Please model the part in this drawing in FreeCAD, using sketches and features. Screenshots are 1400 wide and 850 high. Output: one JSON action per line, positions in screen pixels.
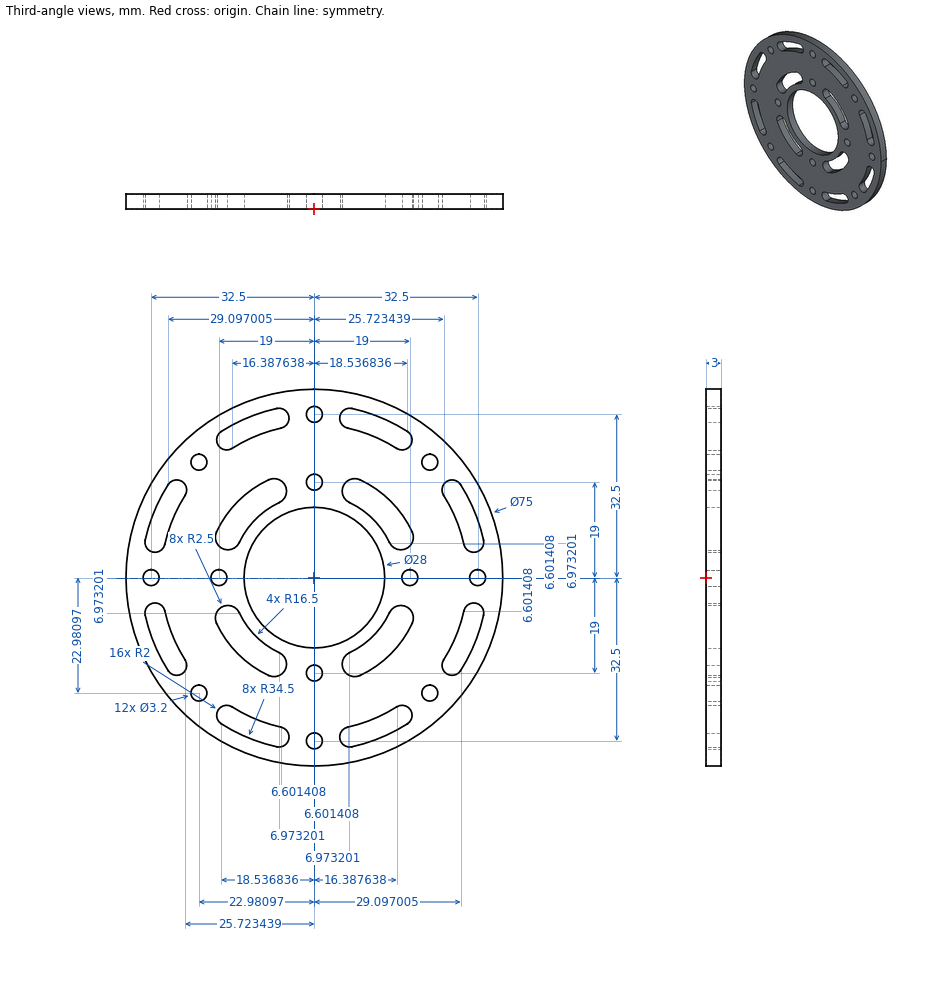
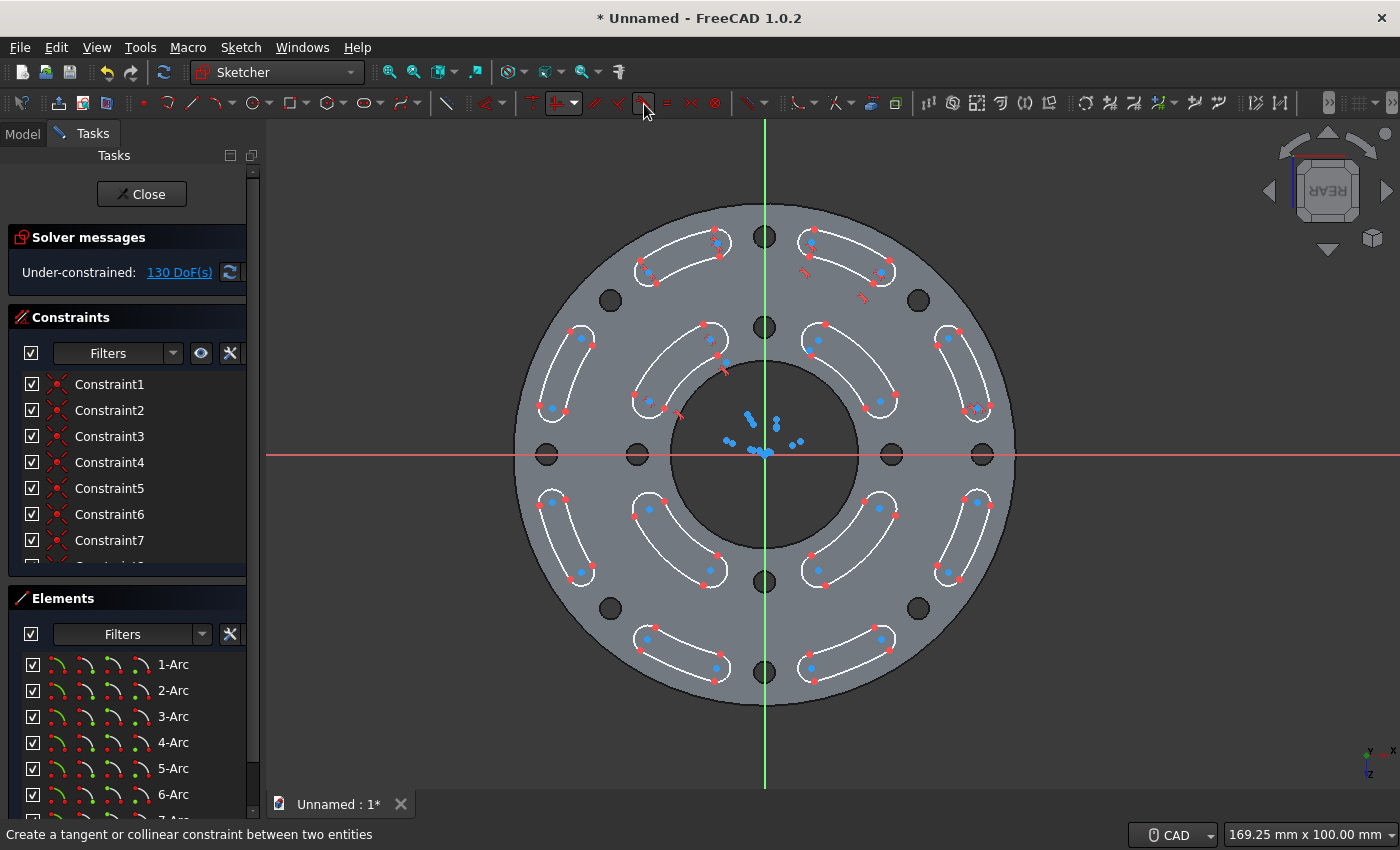
{"action": "left_click", "coordinate": [984, 382]}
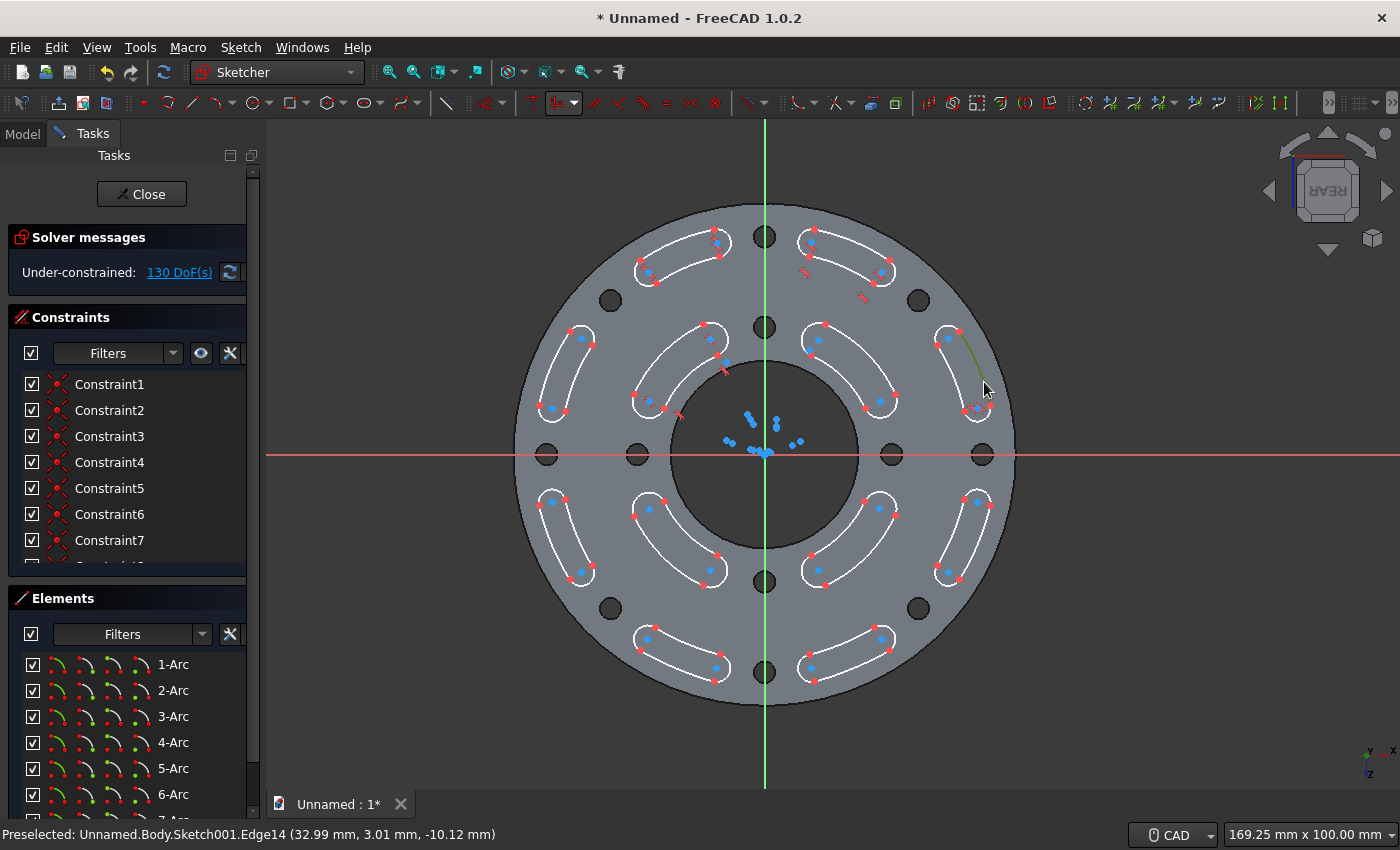
{"action": "left_click", "coordinate": [949, 326]}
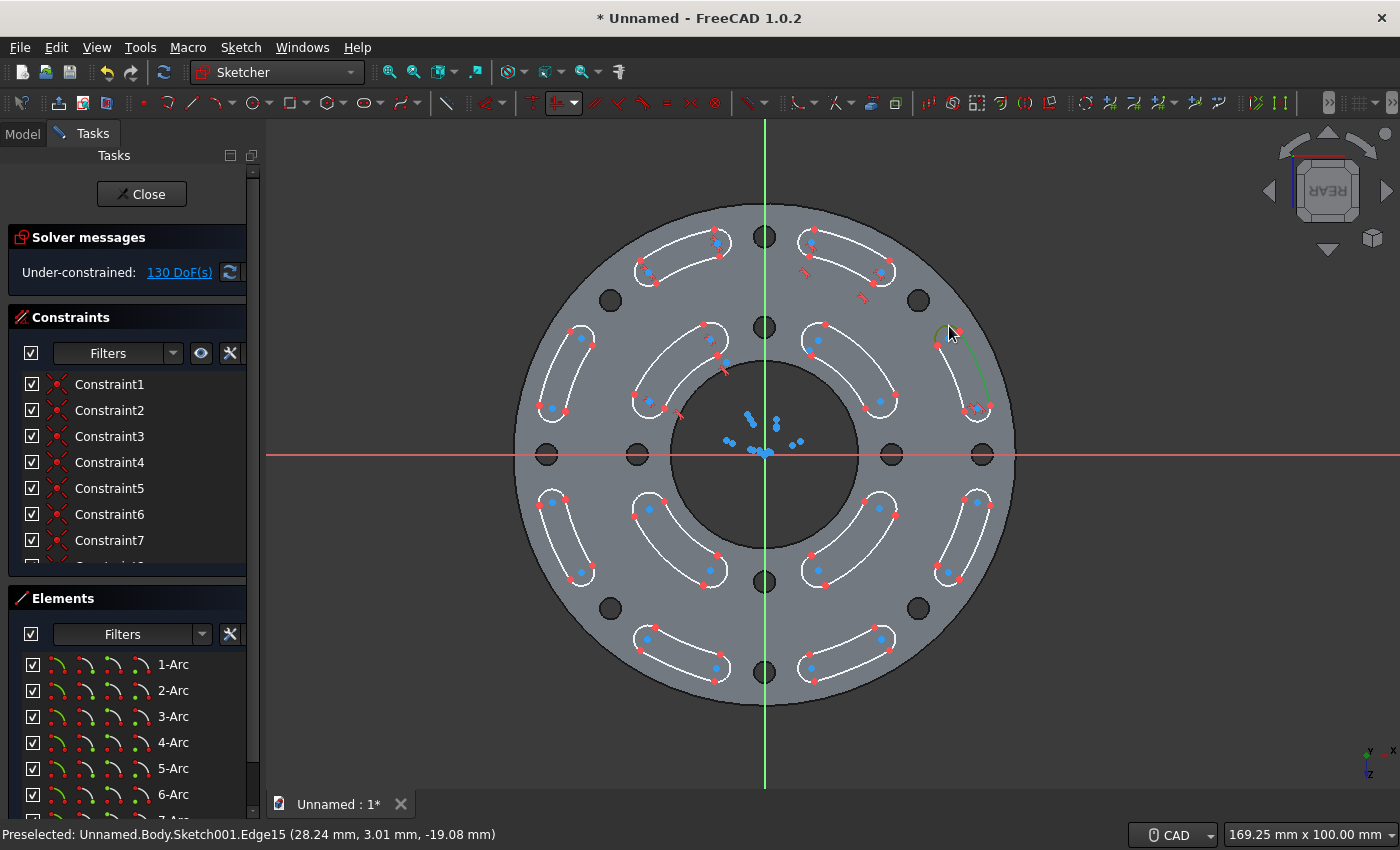
{"action": "left_click", "coordinate": [644, 104]}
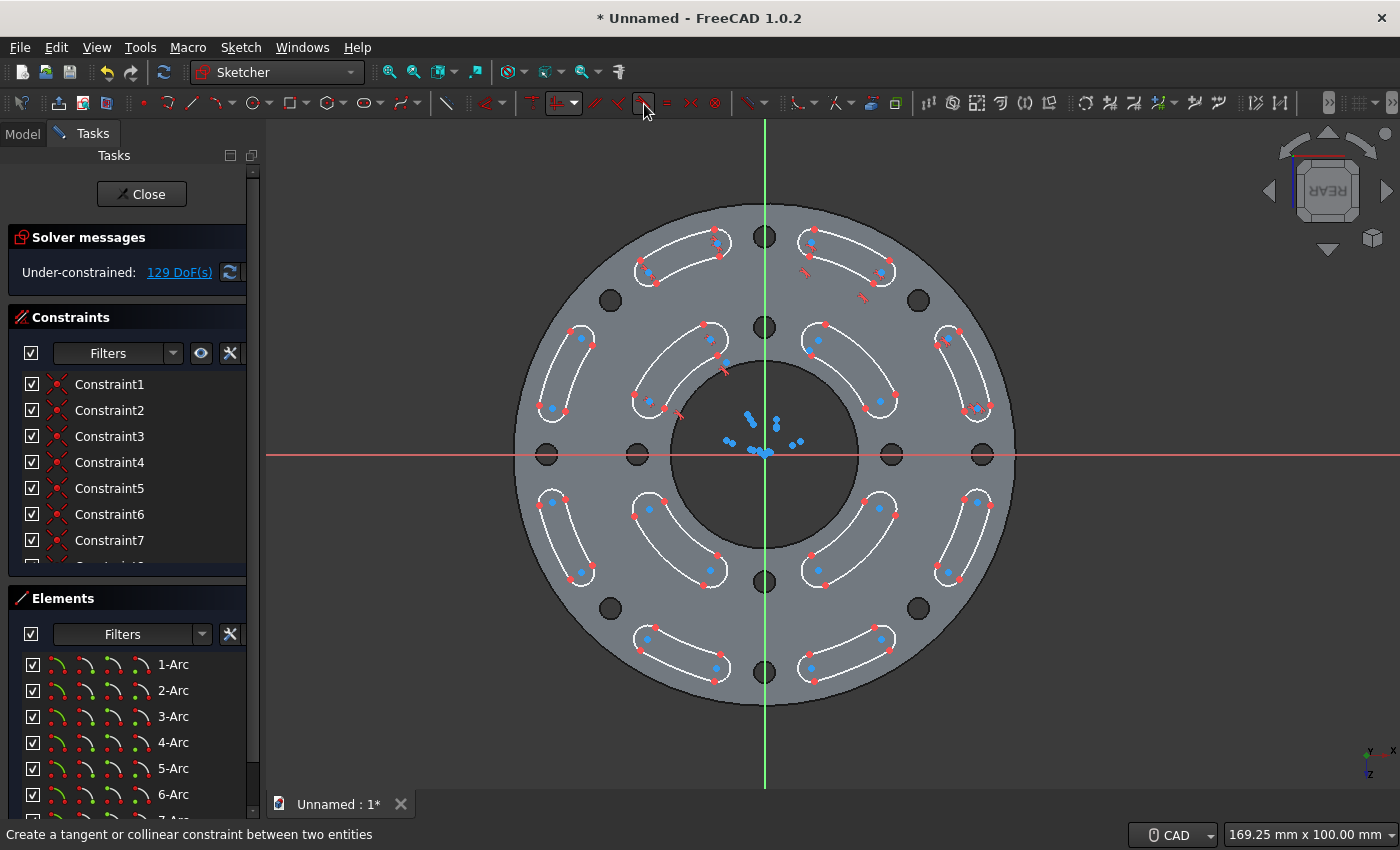
{"action": "left_click", "coordinate": [949, 326]}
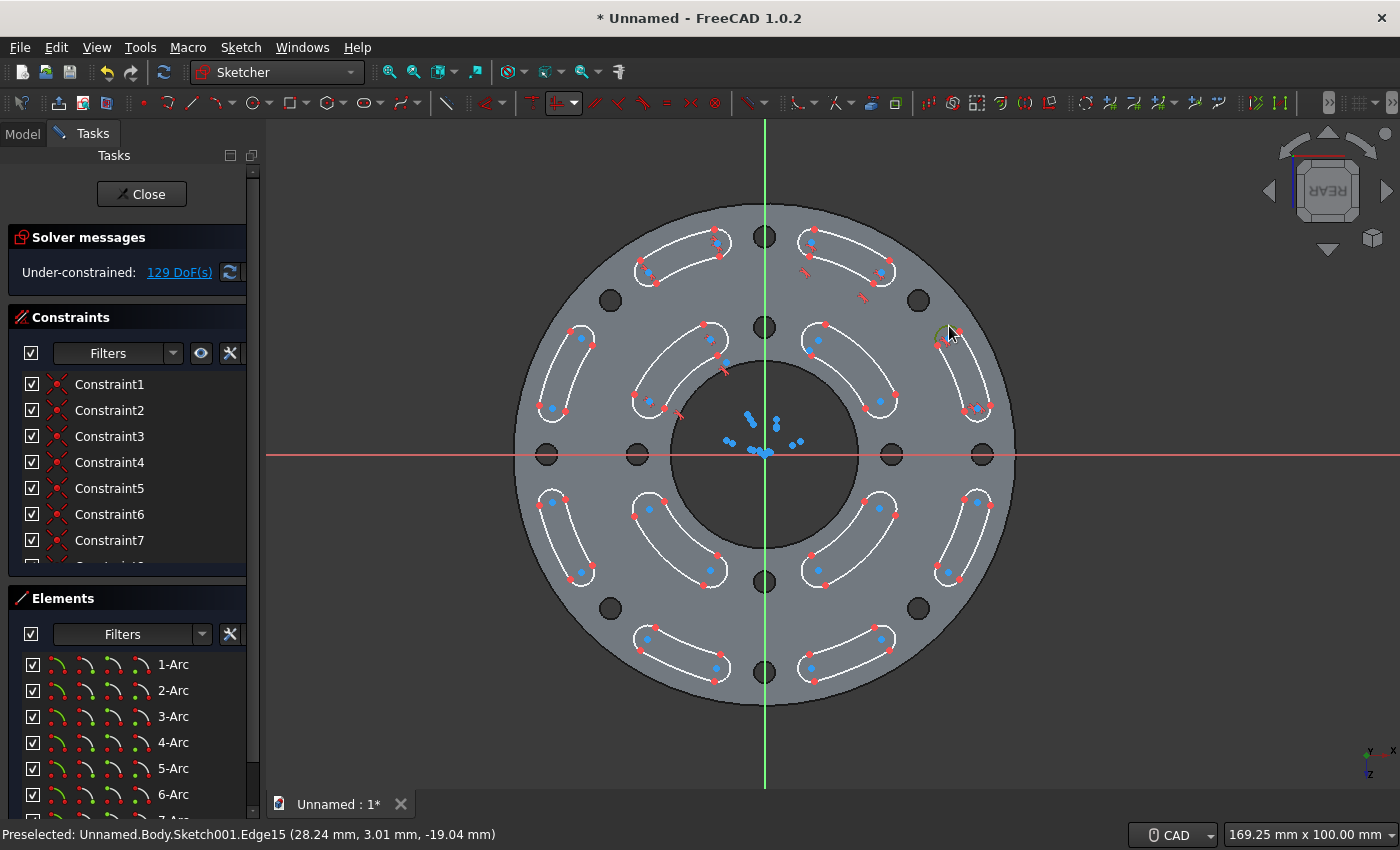
{"action": "left_click", "coordinate": [959, 390]}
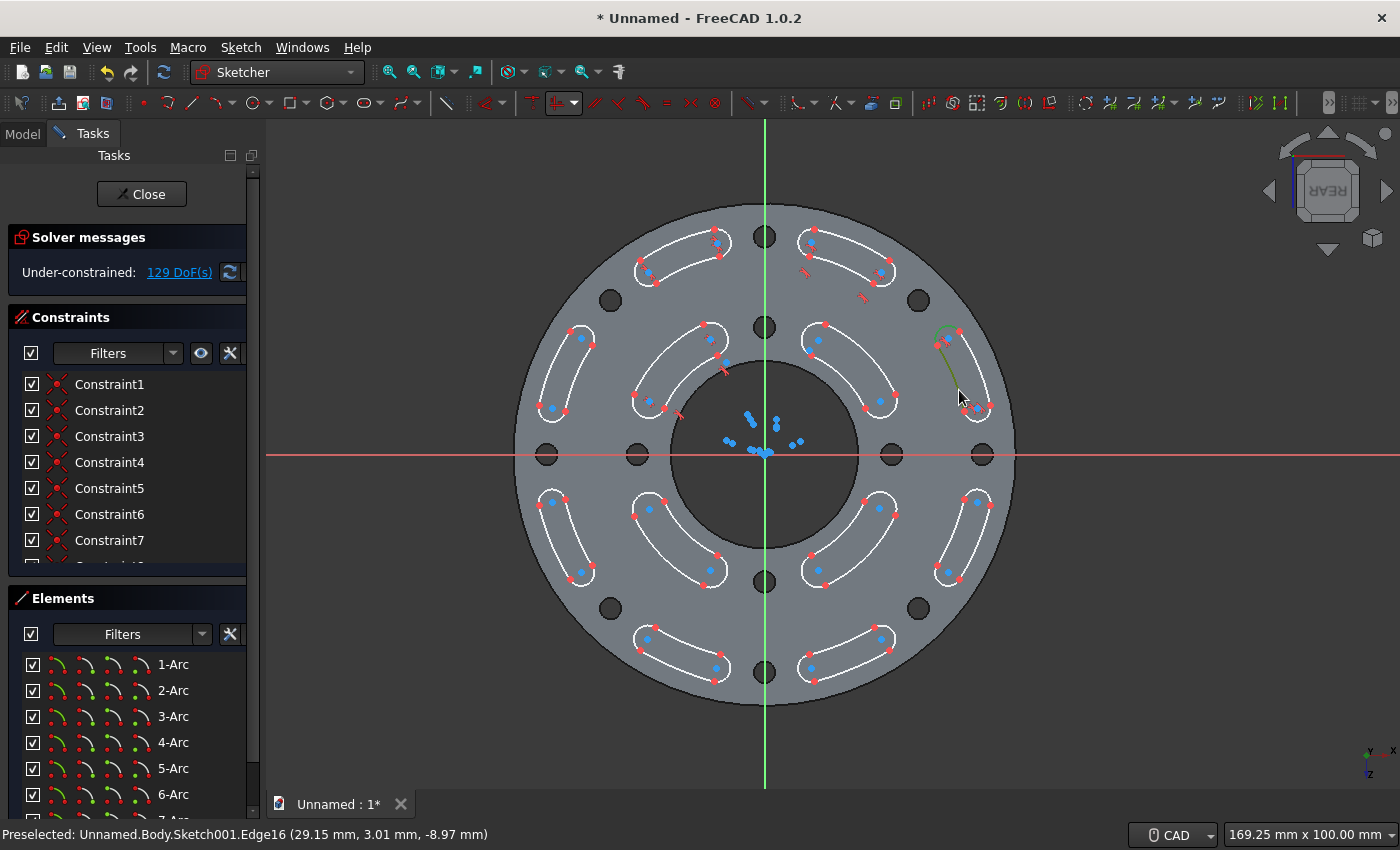
{"action": "left_click", "coordinate": [644, 104]}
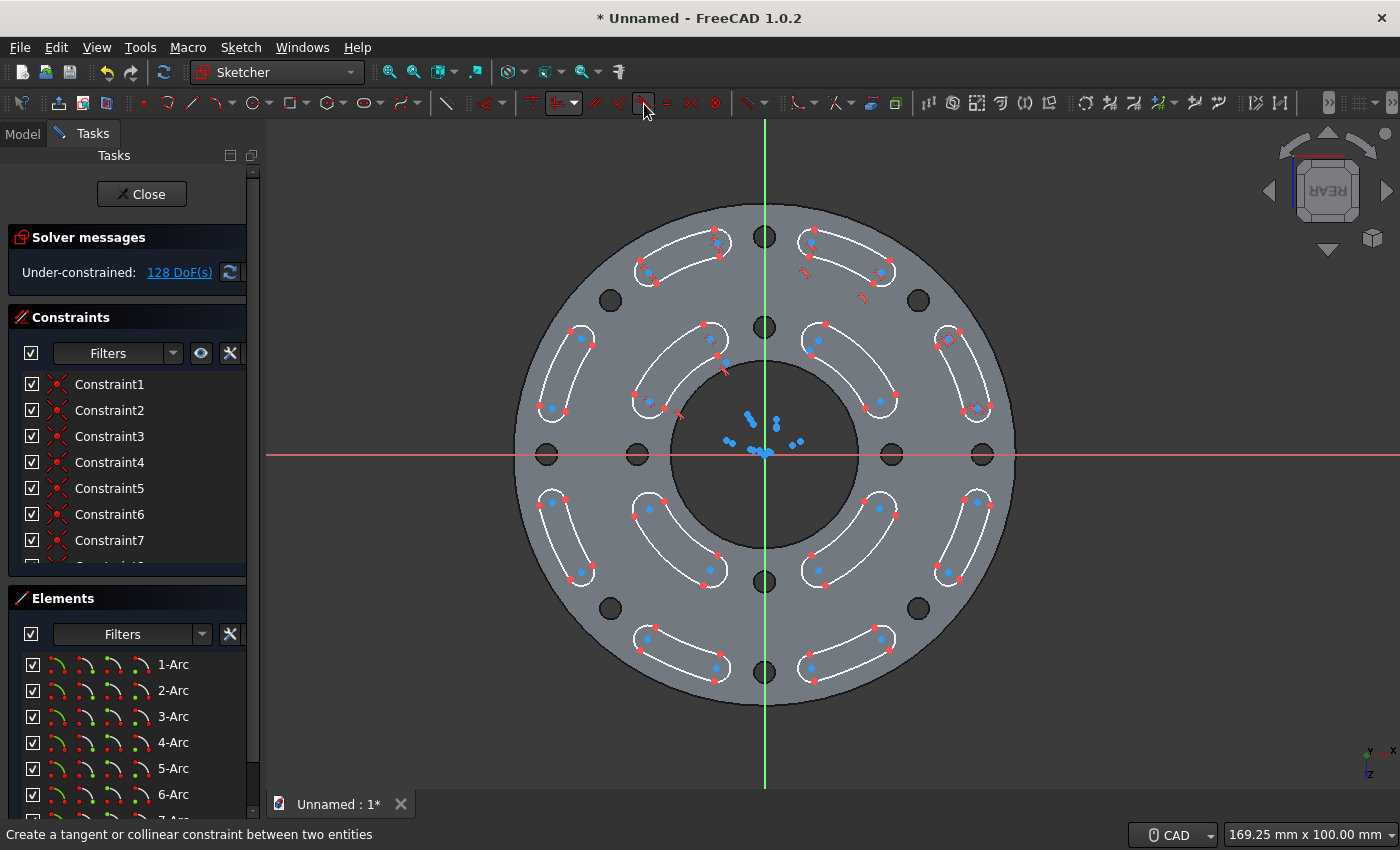
{"action": "left_click", "coordinate": [947, 547]}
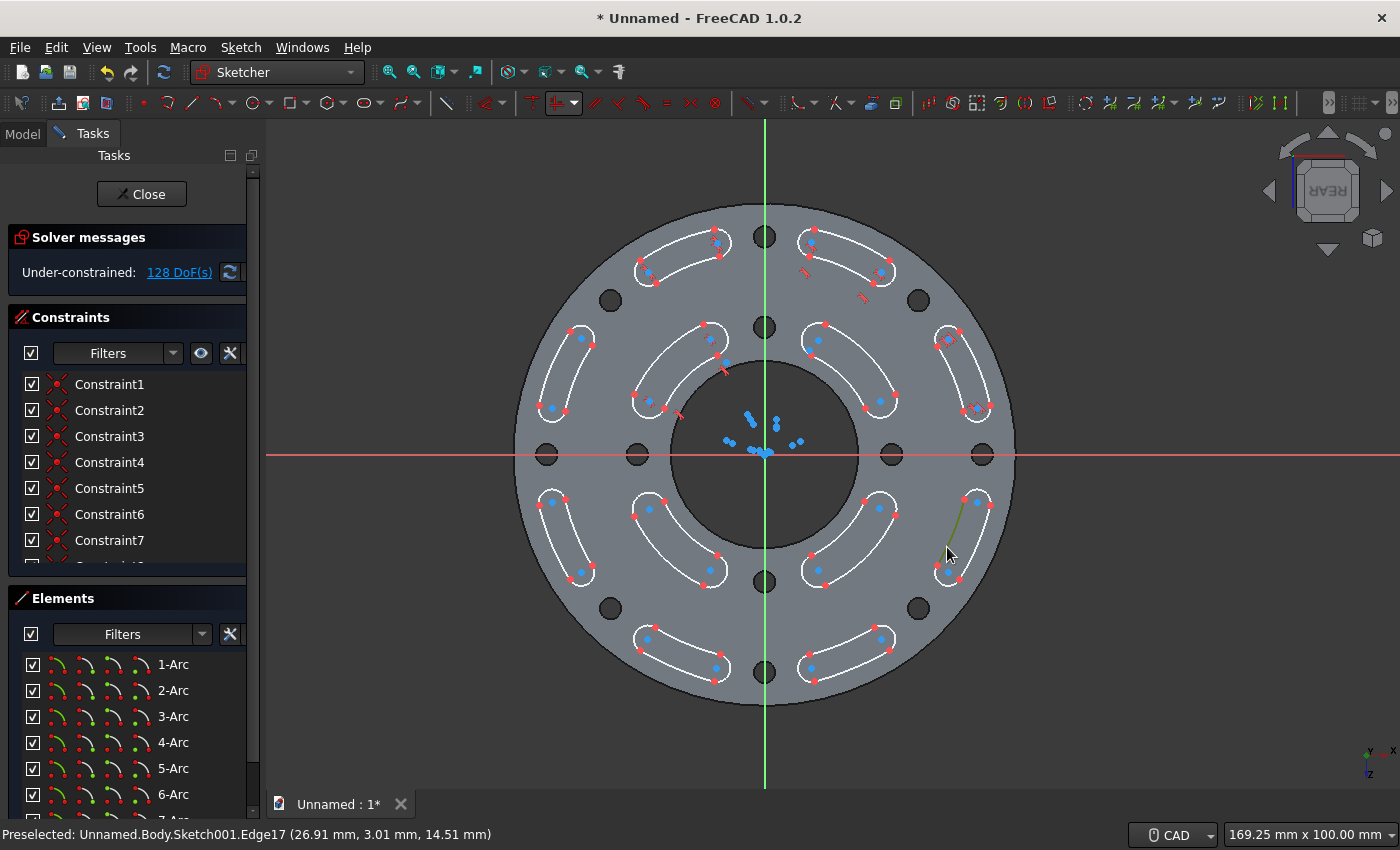
{"action": "left_click", "coordinate": [936, 577]}